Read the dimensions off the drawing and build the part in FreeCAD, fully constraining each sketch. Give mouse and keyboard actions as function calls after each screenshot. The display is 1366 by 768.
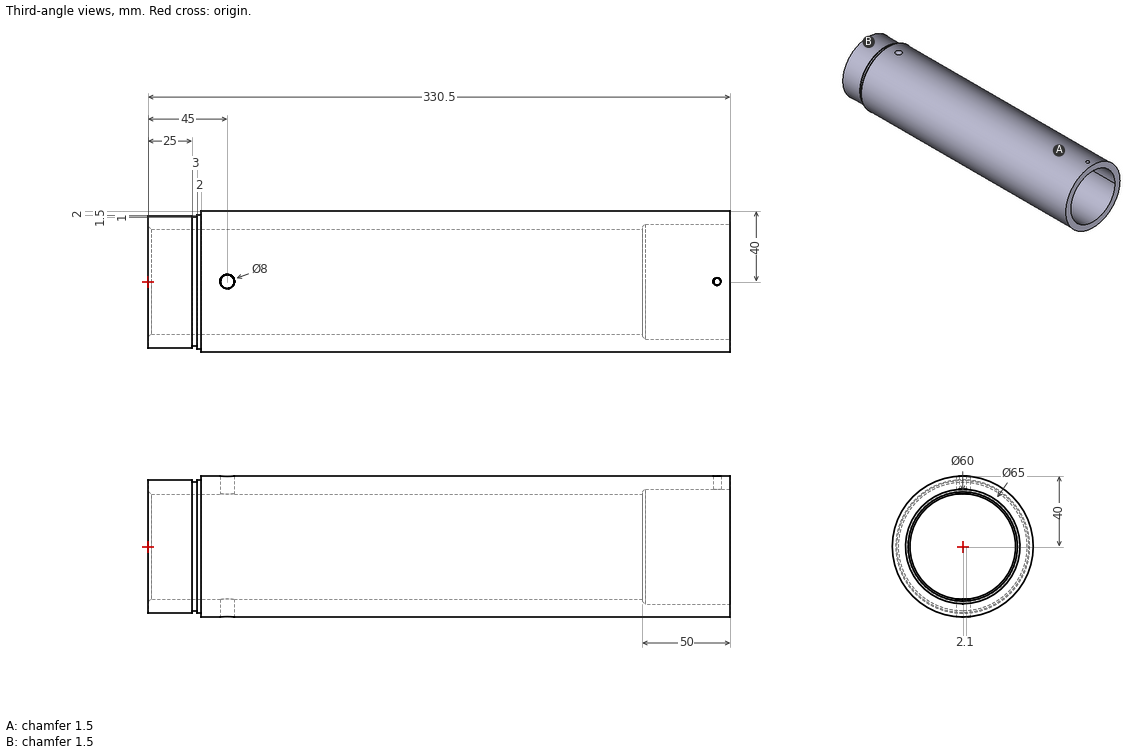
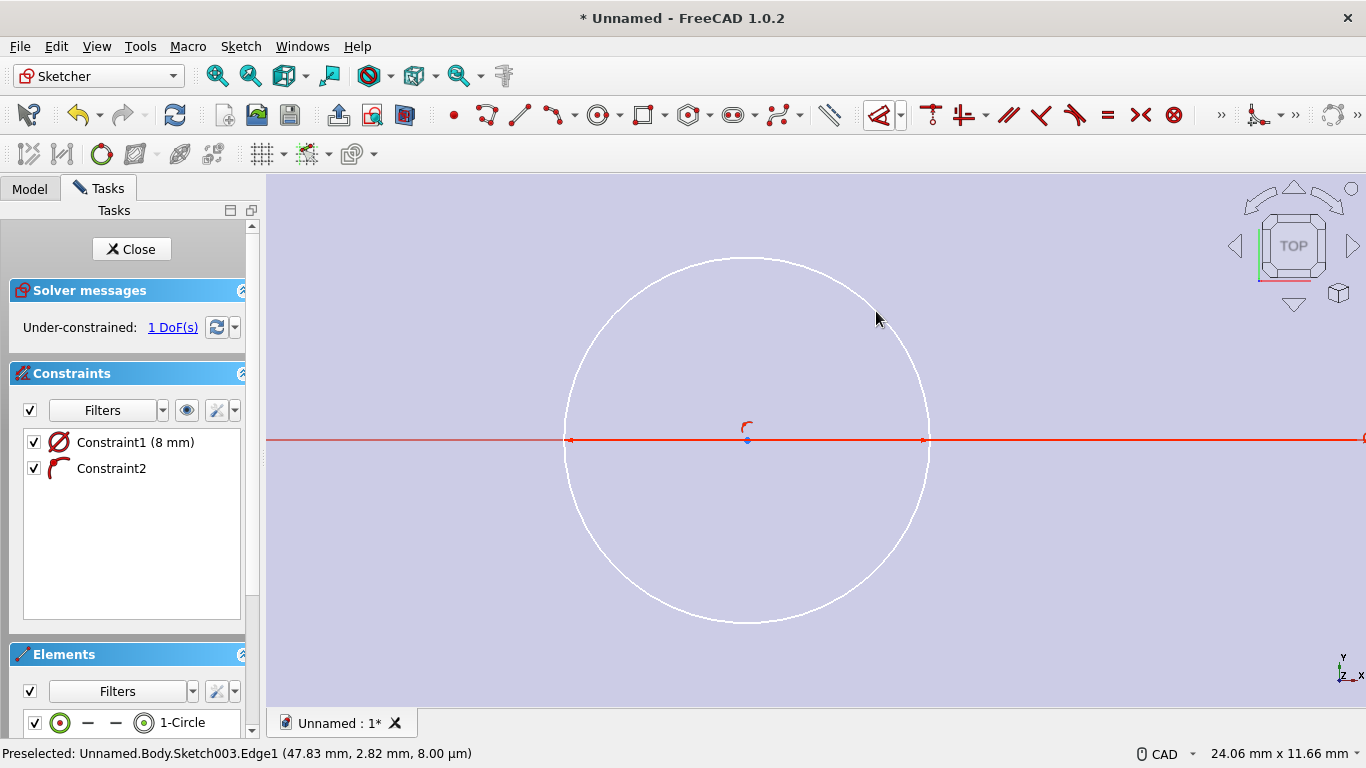
click(747, 440)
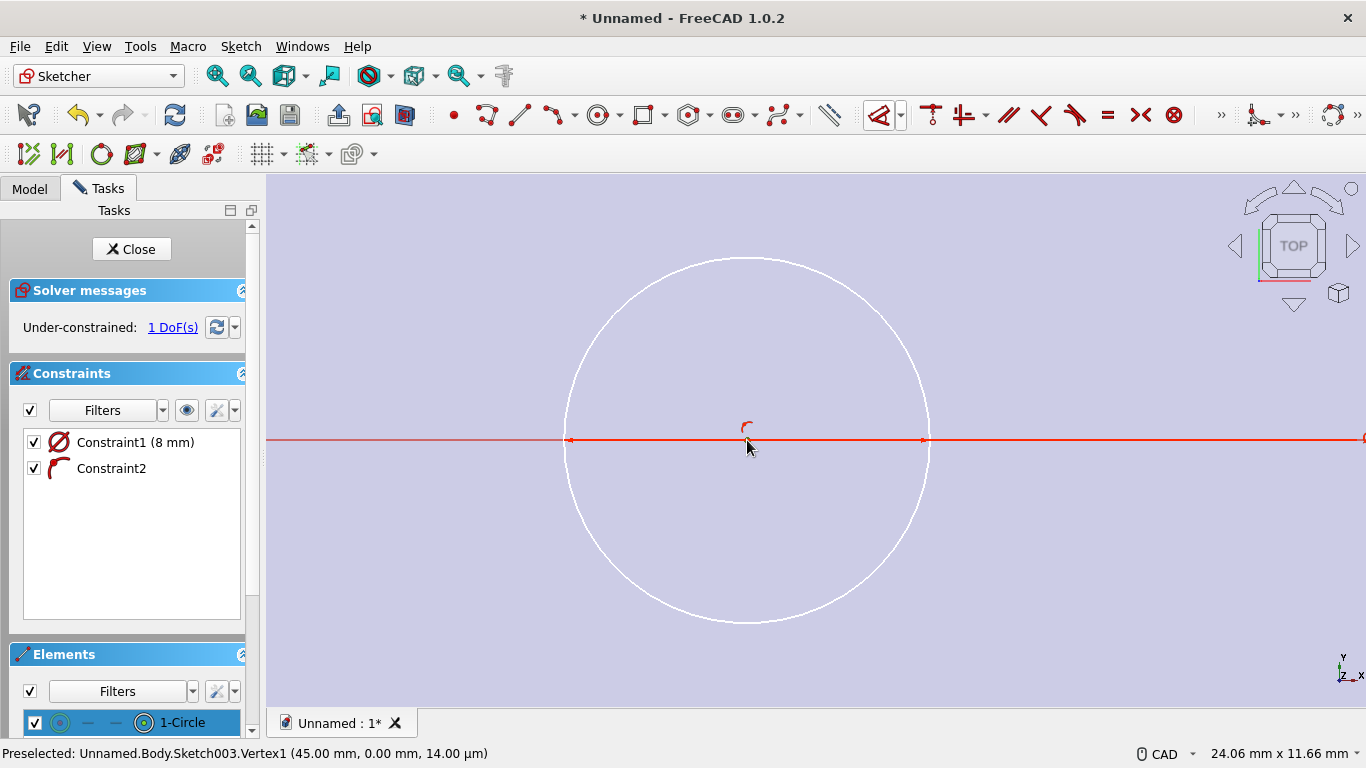
click(900, 116)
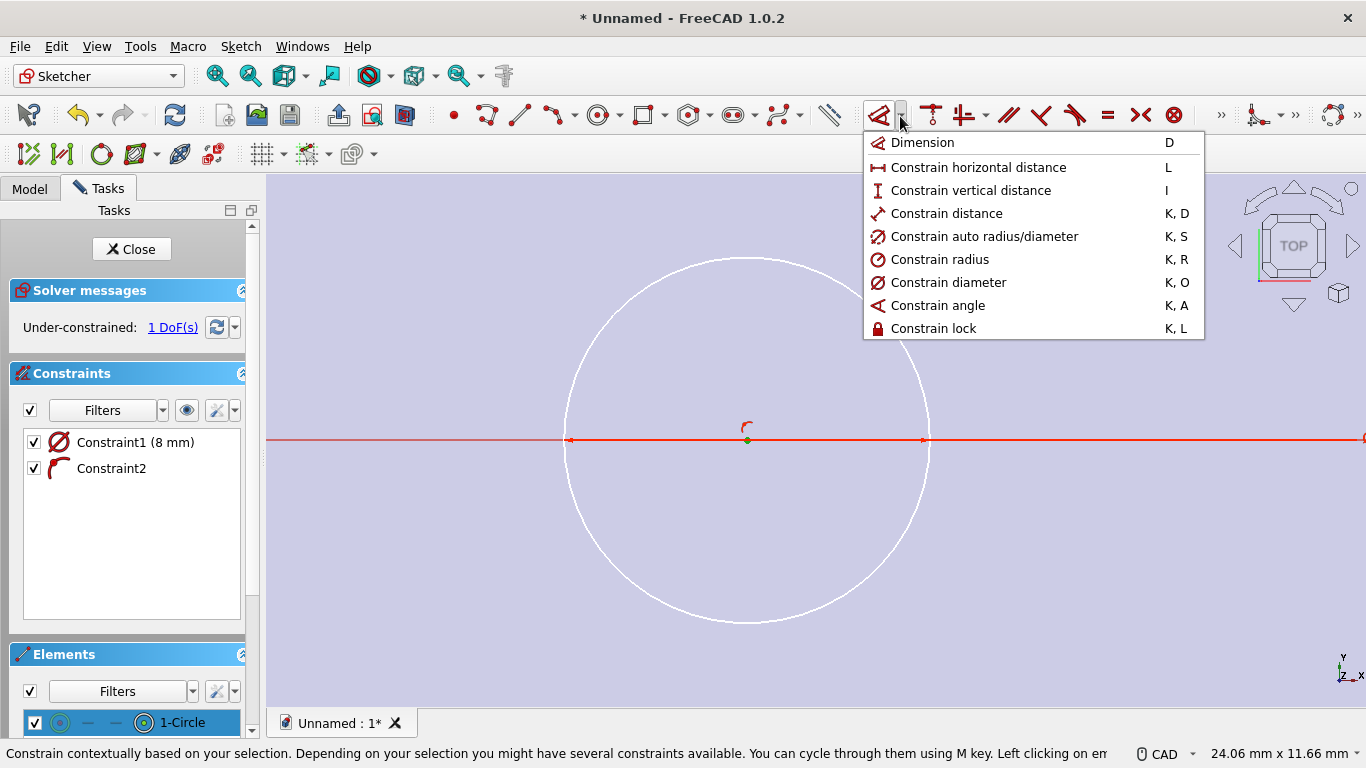
click(1034, 168)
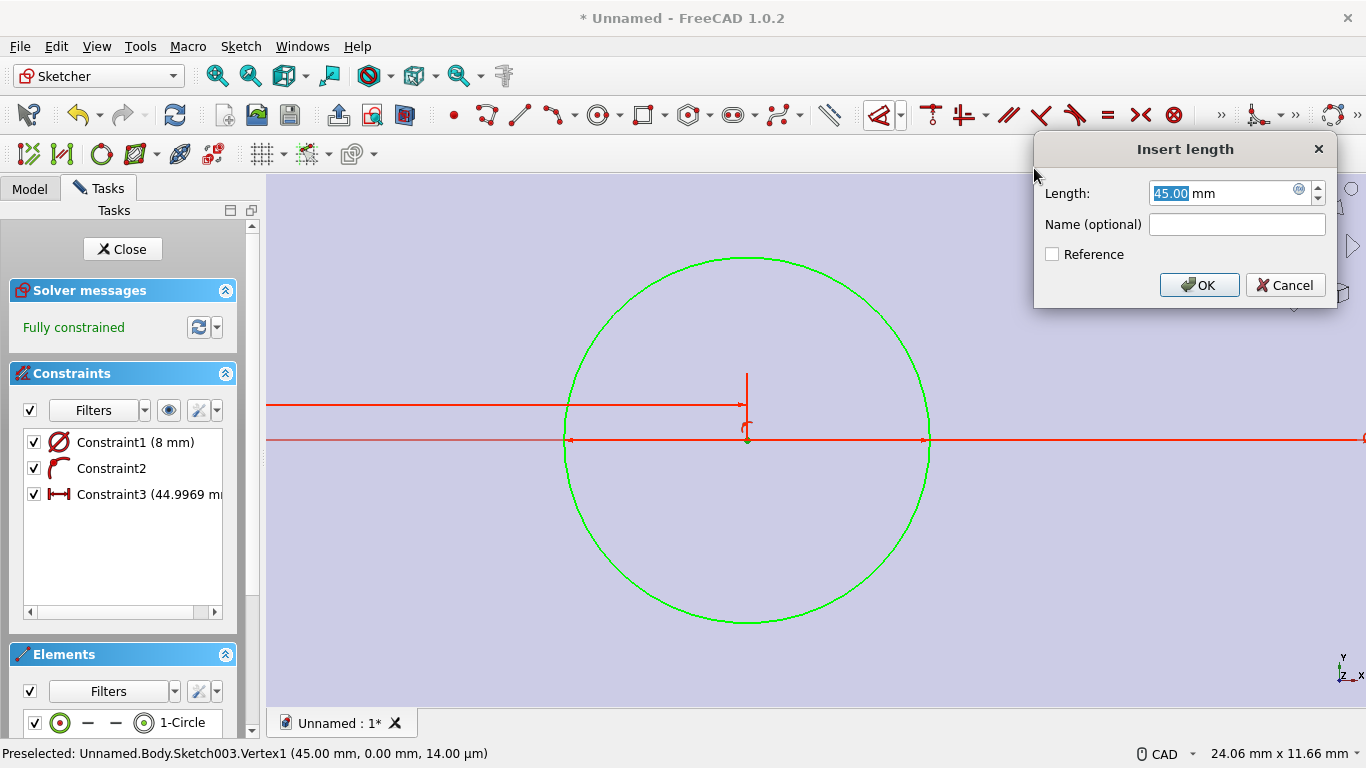
text(45)
key(Return)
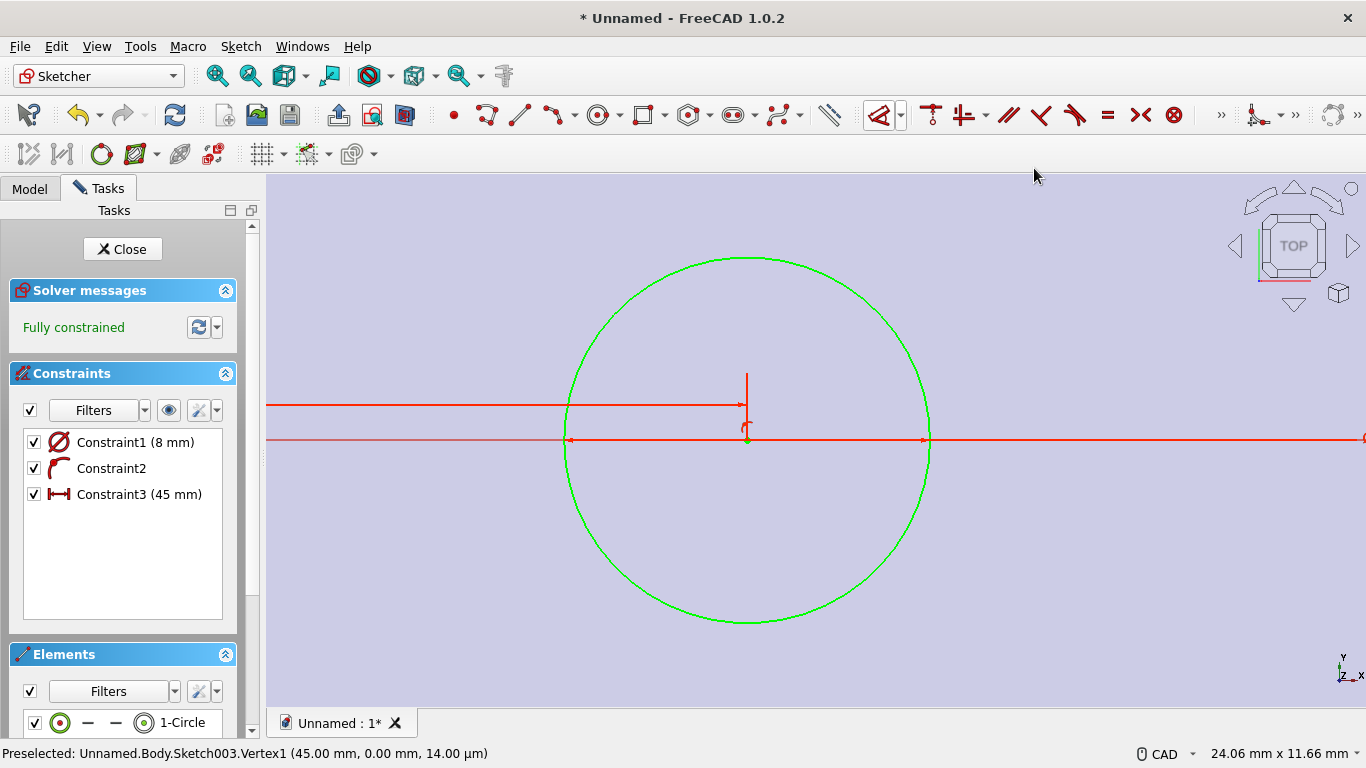
click(123, 249)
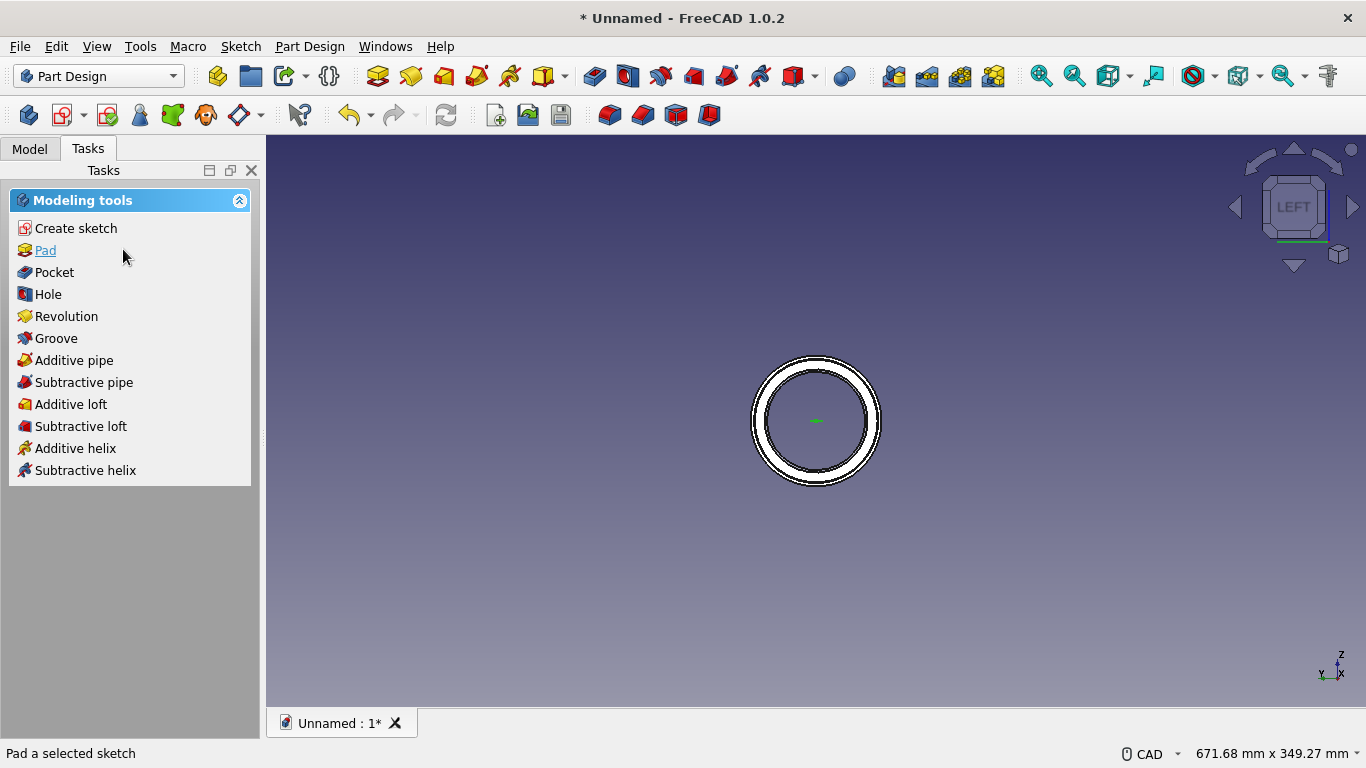
click(595, 76)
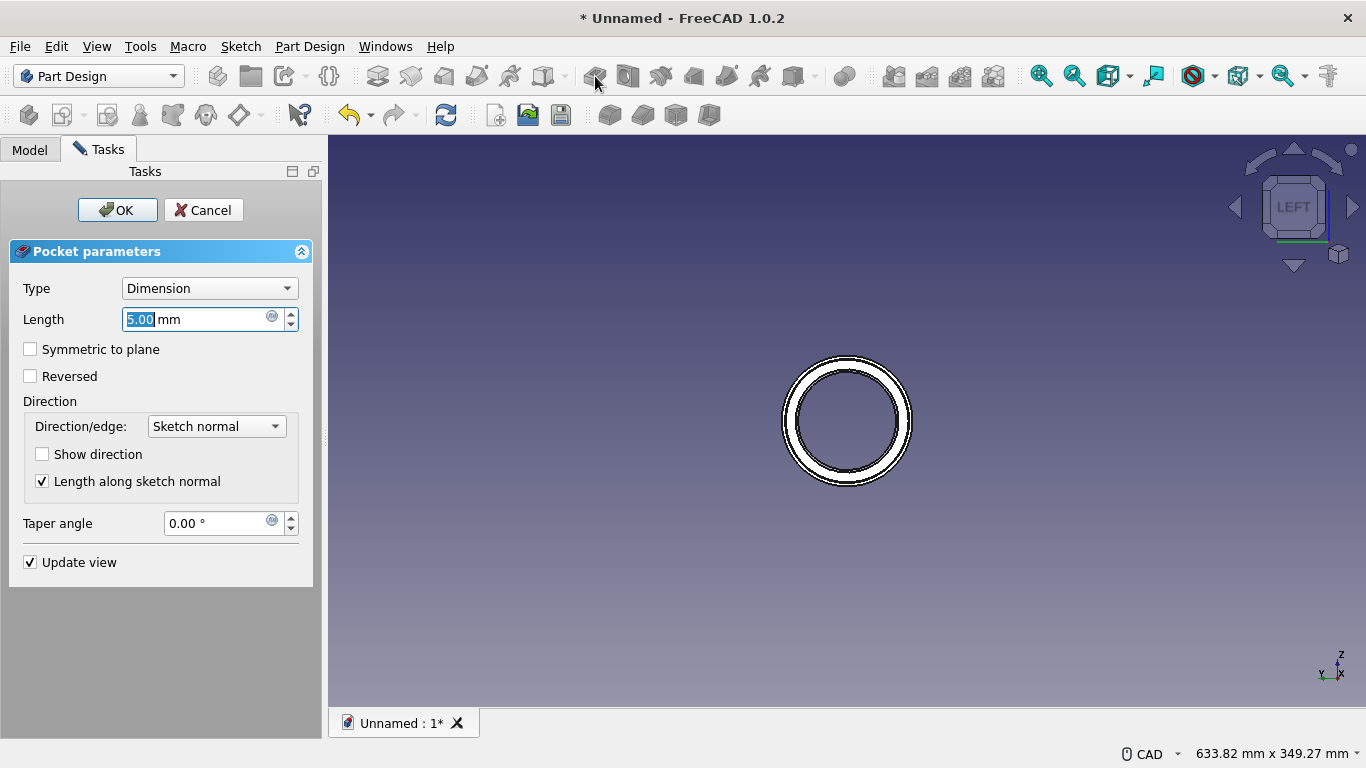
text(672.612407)
key(Tab)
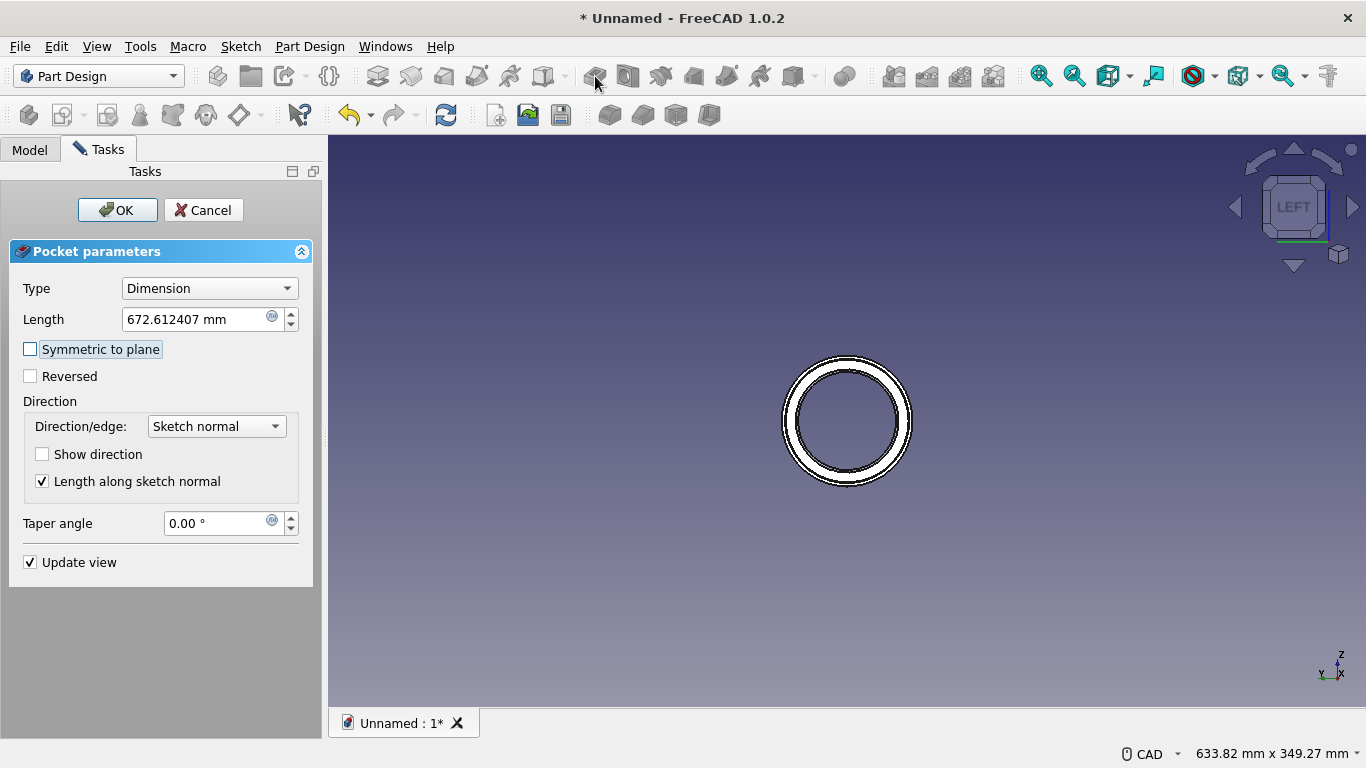
click(31, 349)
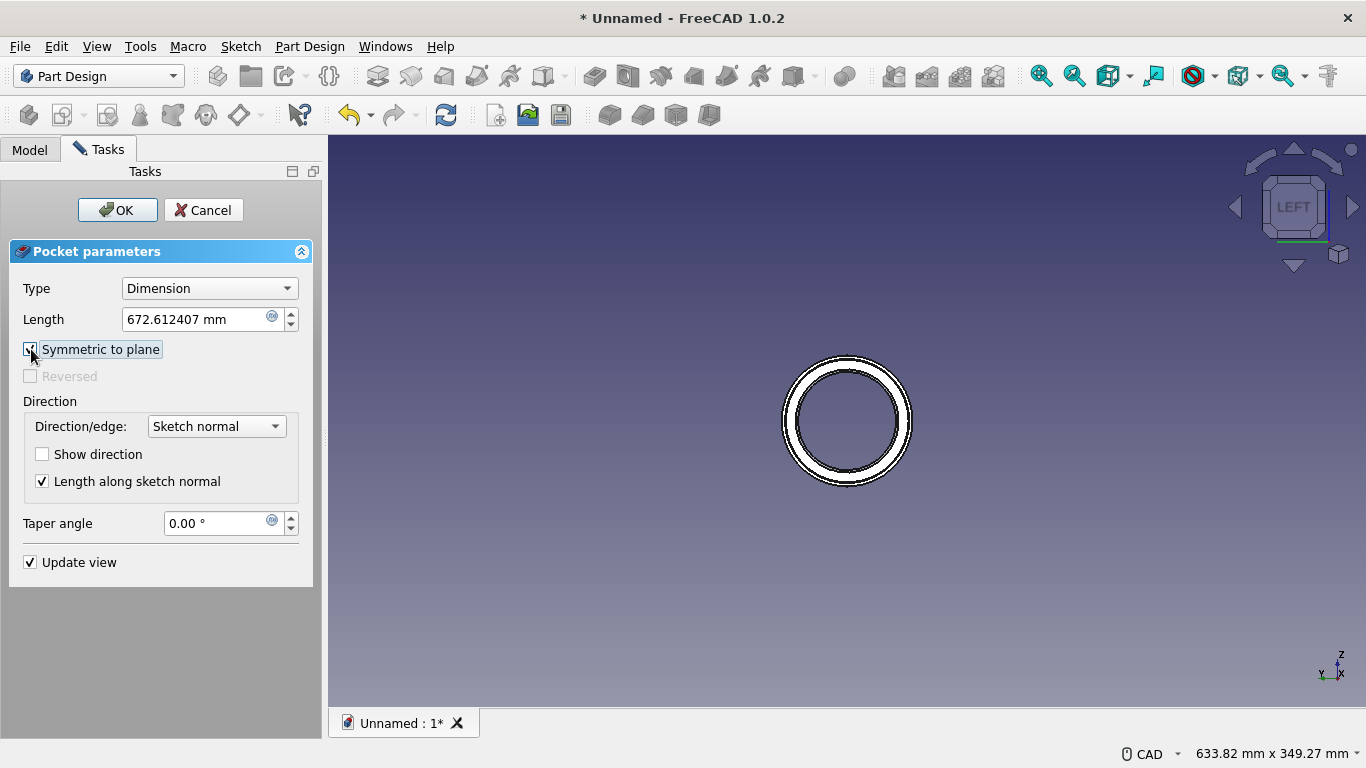
click(118, 210)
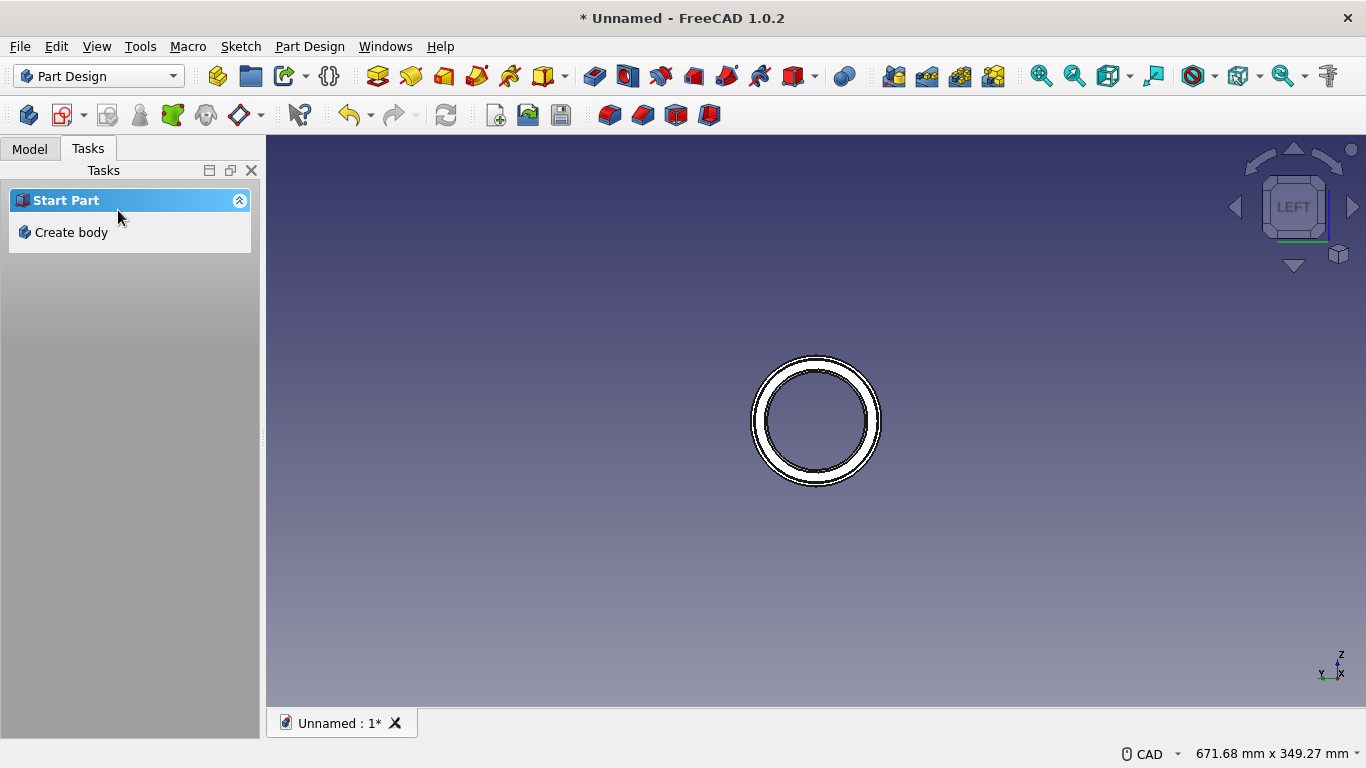
click(1042, 76)